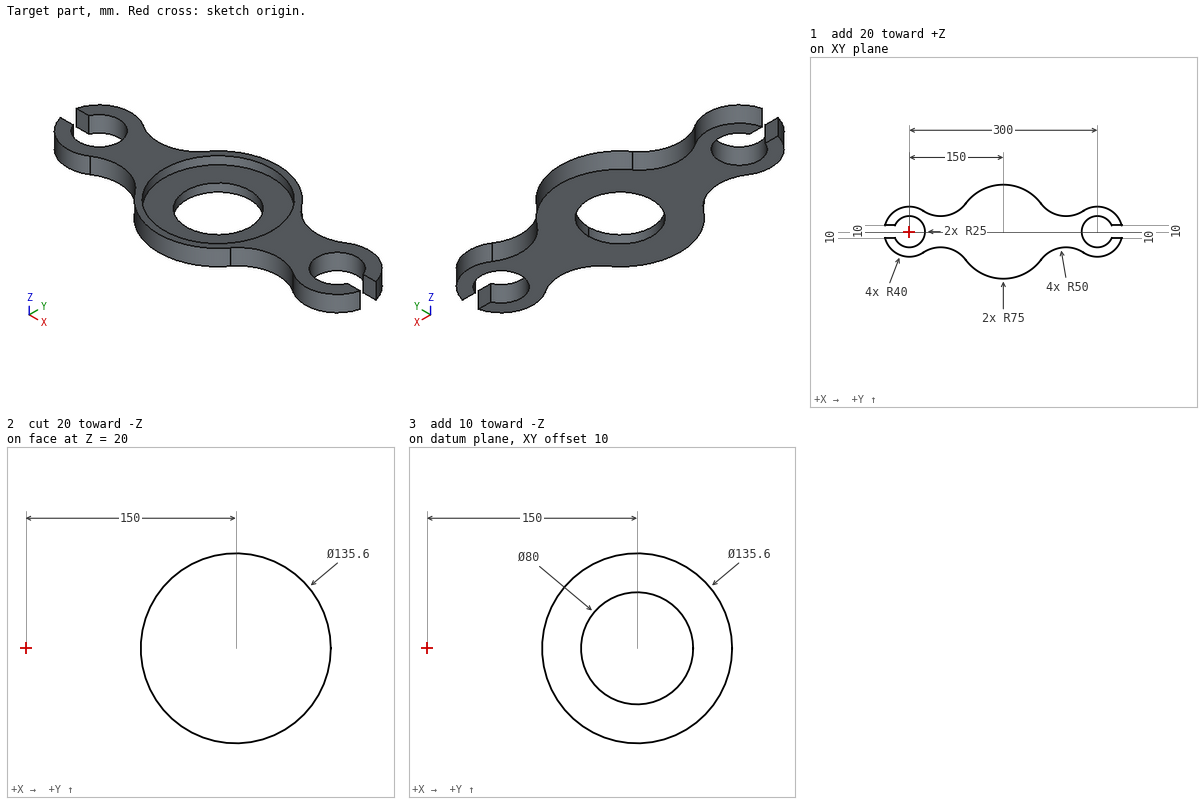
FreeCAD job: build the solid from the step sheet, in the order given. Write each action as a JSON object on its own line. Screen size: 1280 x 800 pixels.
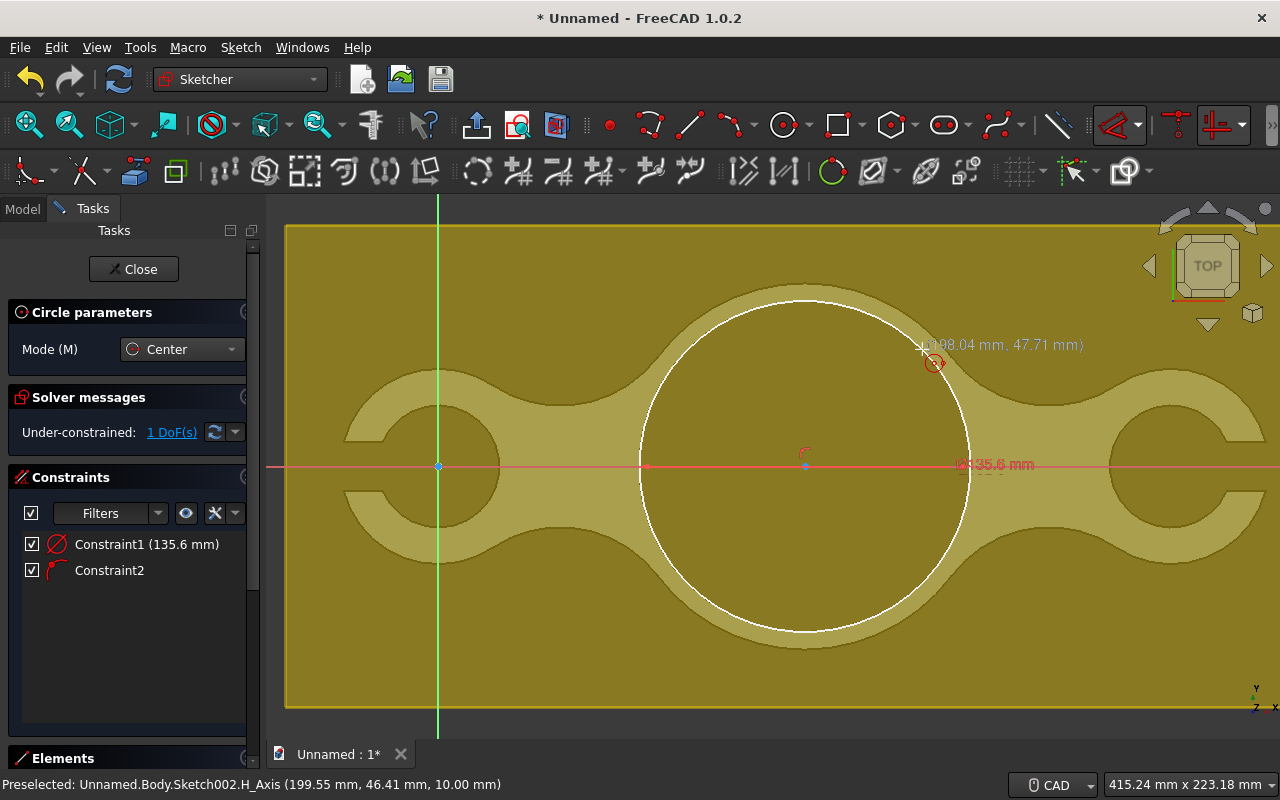
{"action": "left_click", "coordinate": [805, 466]}
{"action": "mouse_move", "coordinate": [874, 397]}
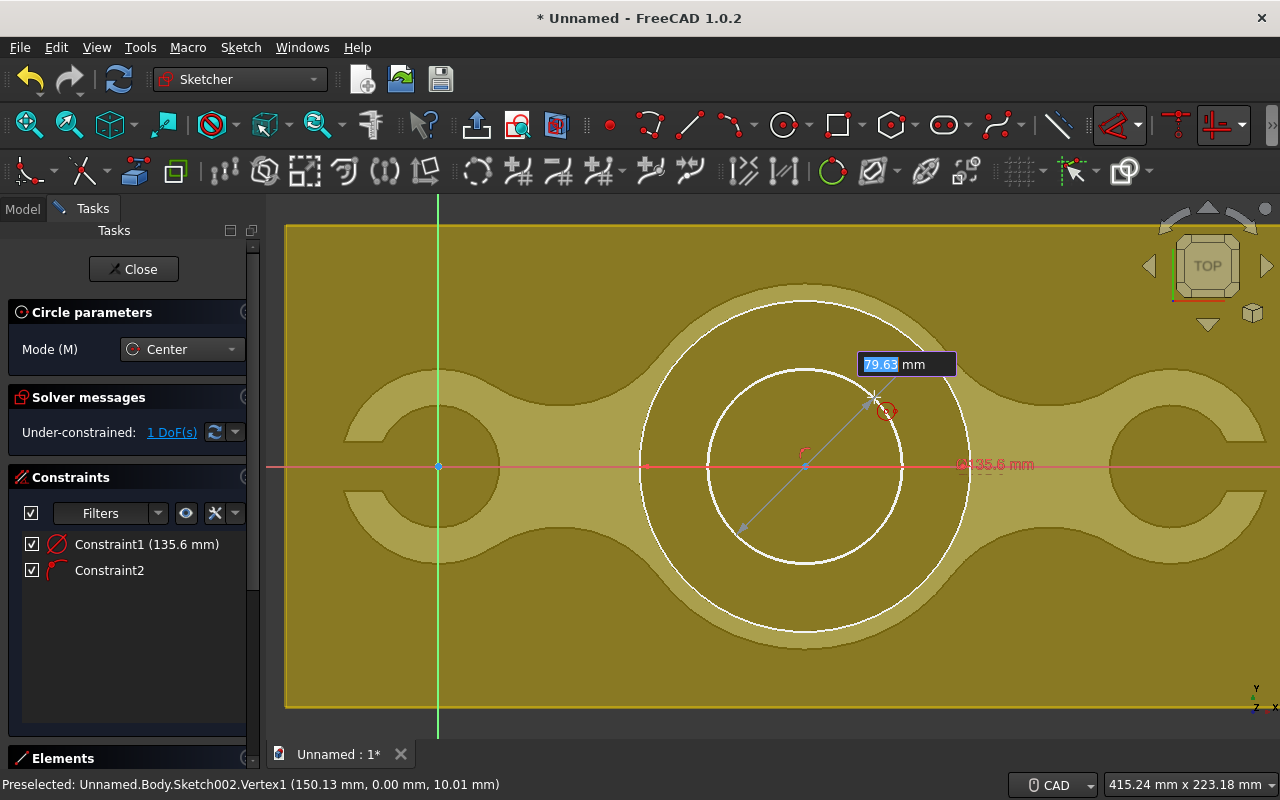
{"action": "type", "text": "80"}
{"action": "key", "text": "Return"}
{"action": "key", "text": "Escape"}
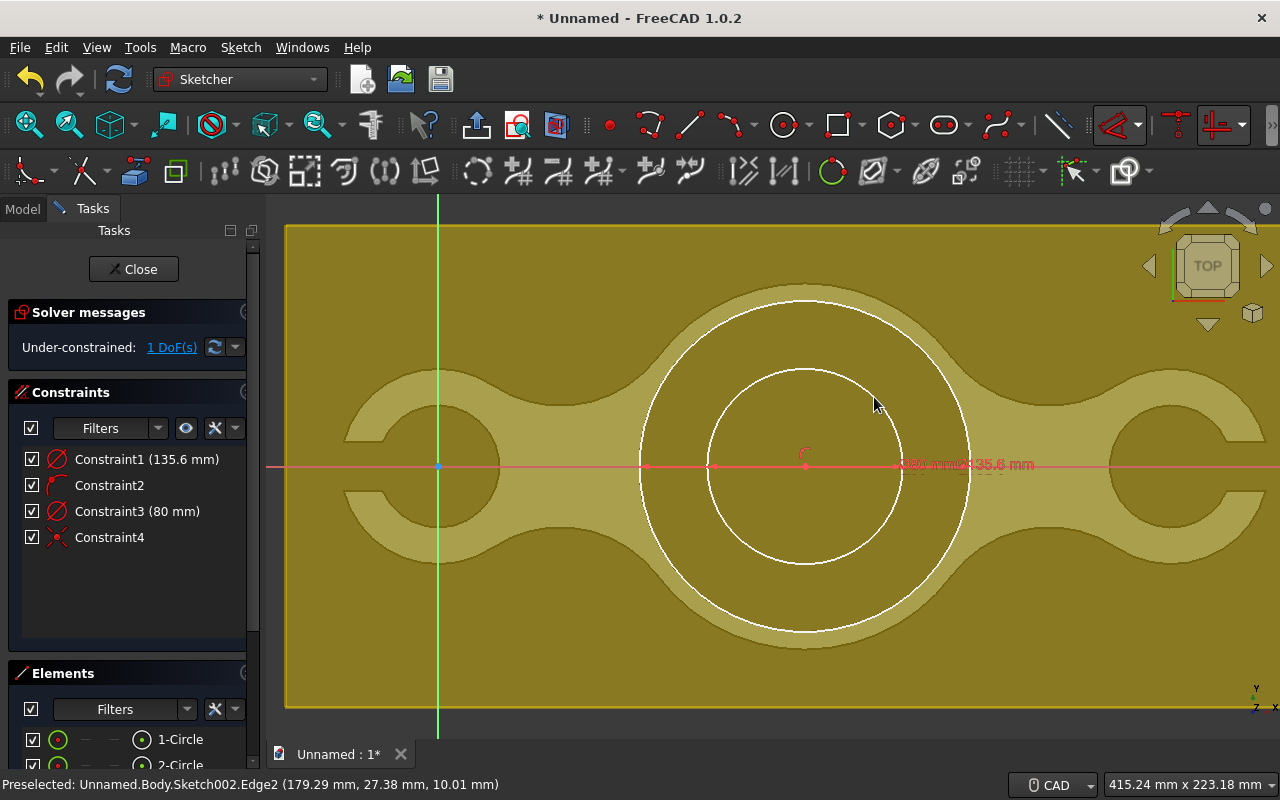
{"action": "left_click", "coordinate": [805, 466]}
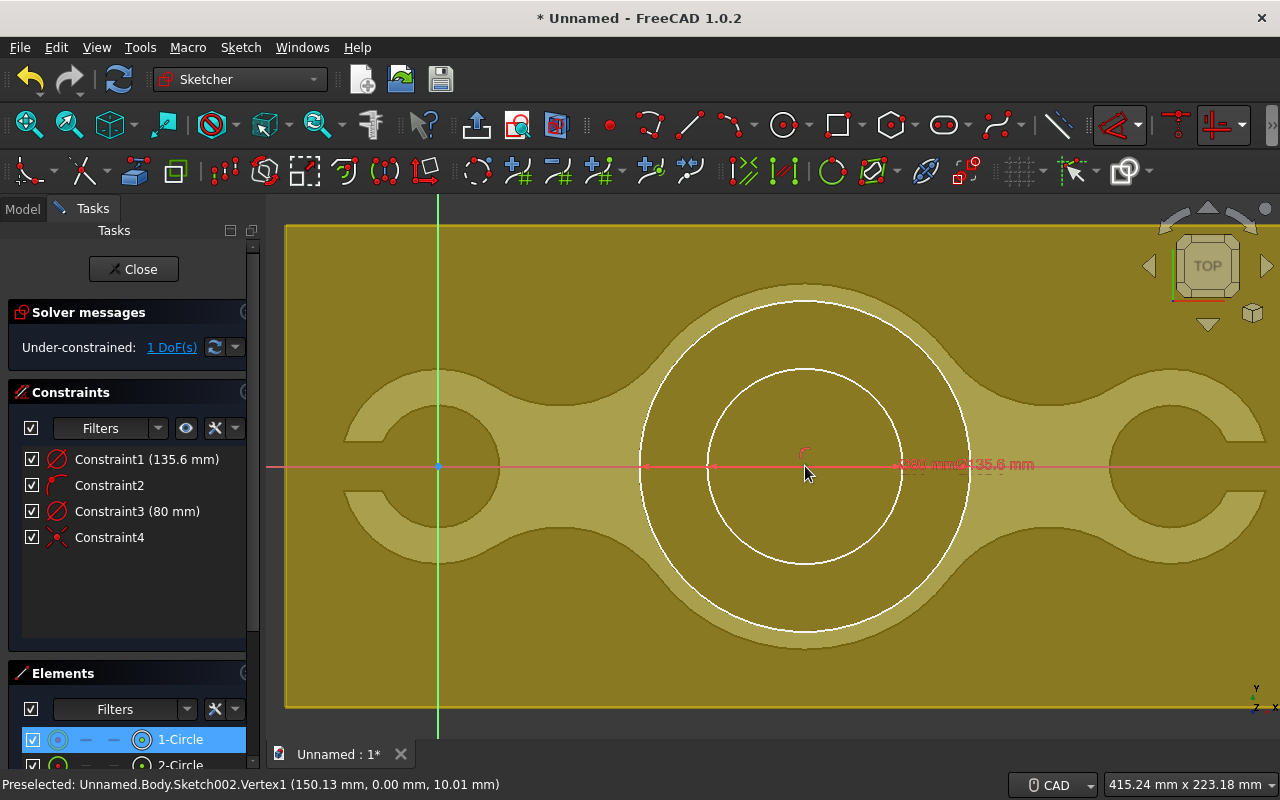
{"action": "key", "text": "l"}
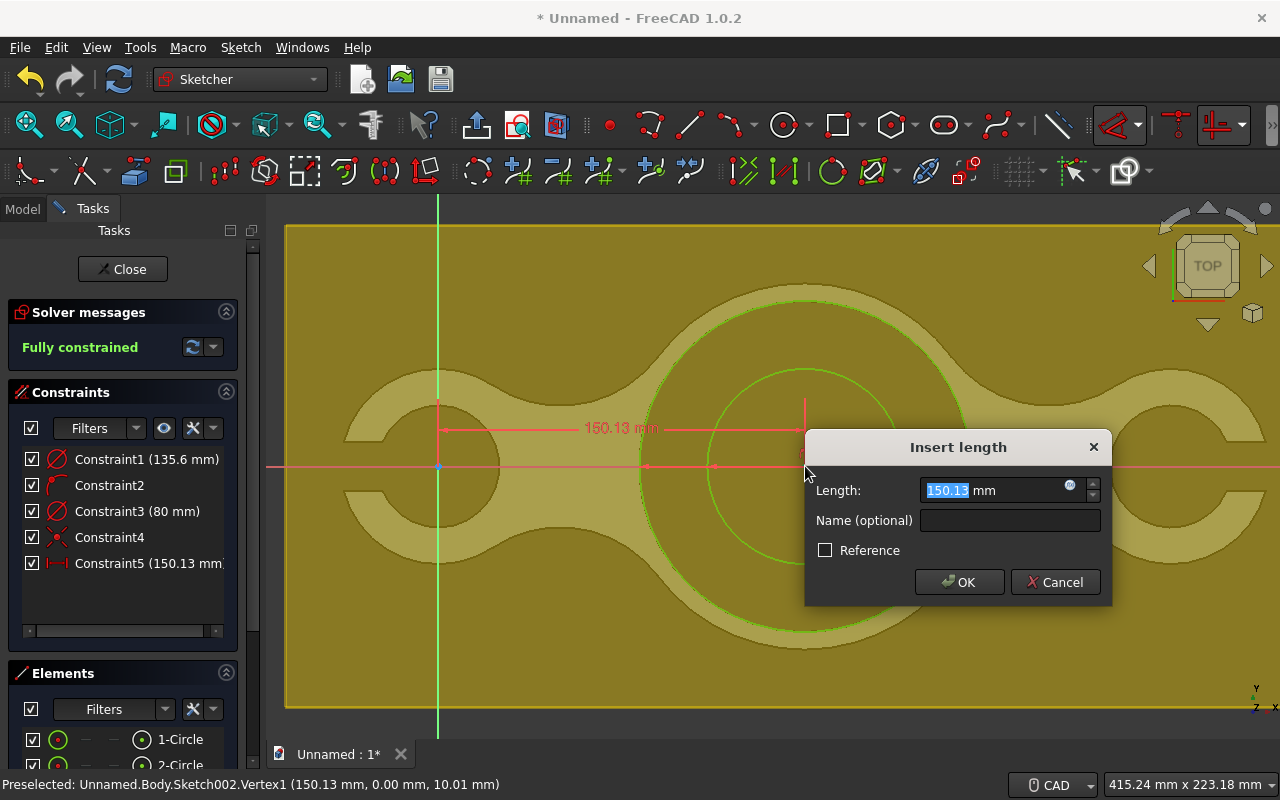
{"action": "type", "text": "150"}
{"action": "key", "text": "Return"}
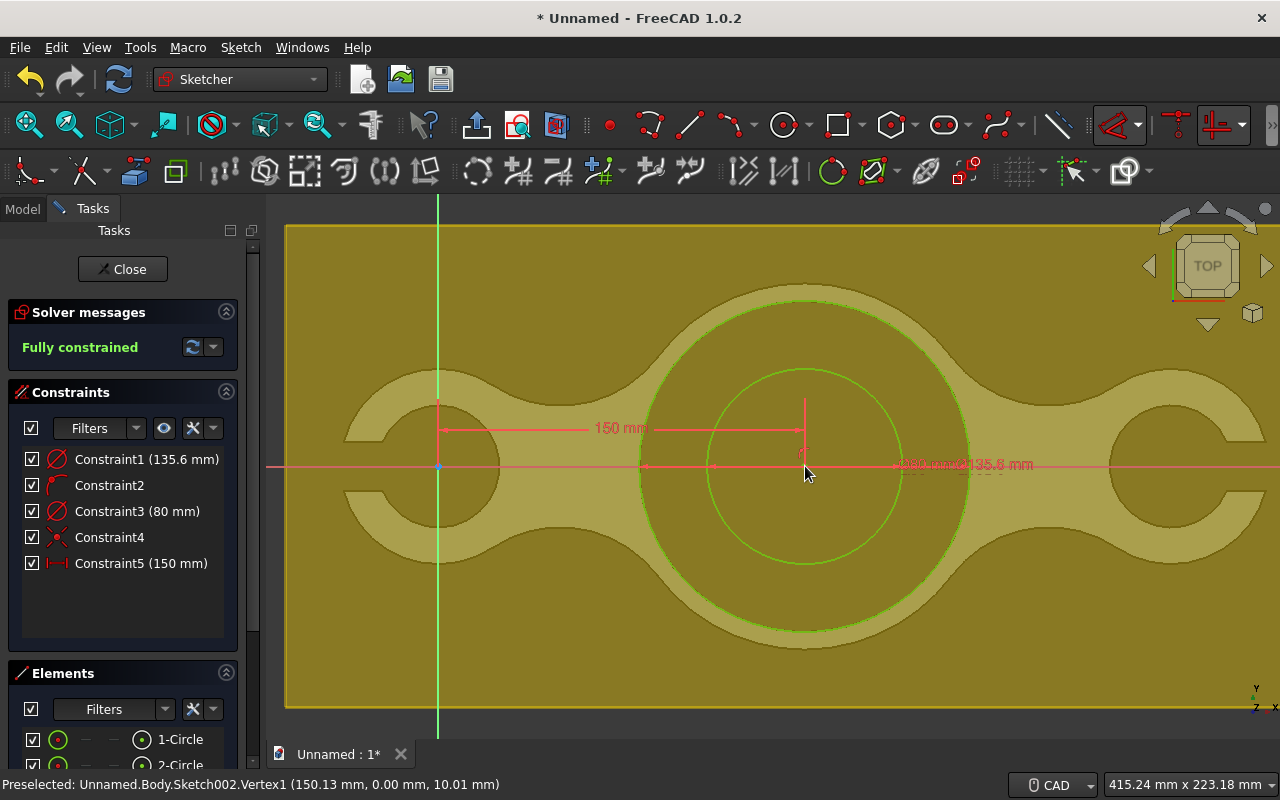
{"action": "left_click", "coordinate": [123, 269]}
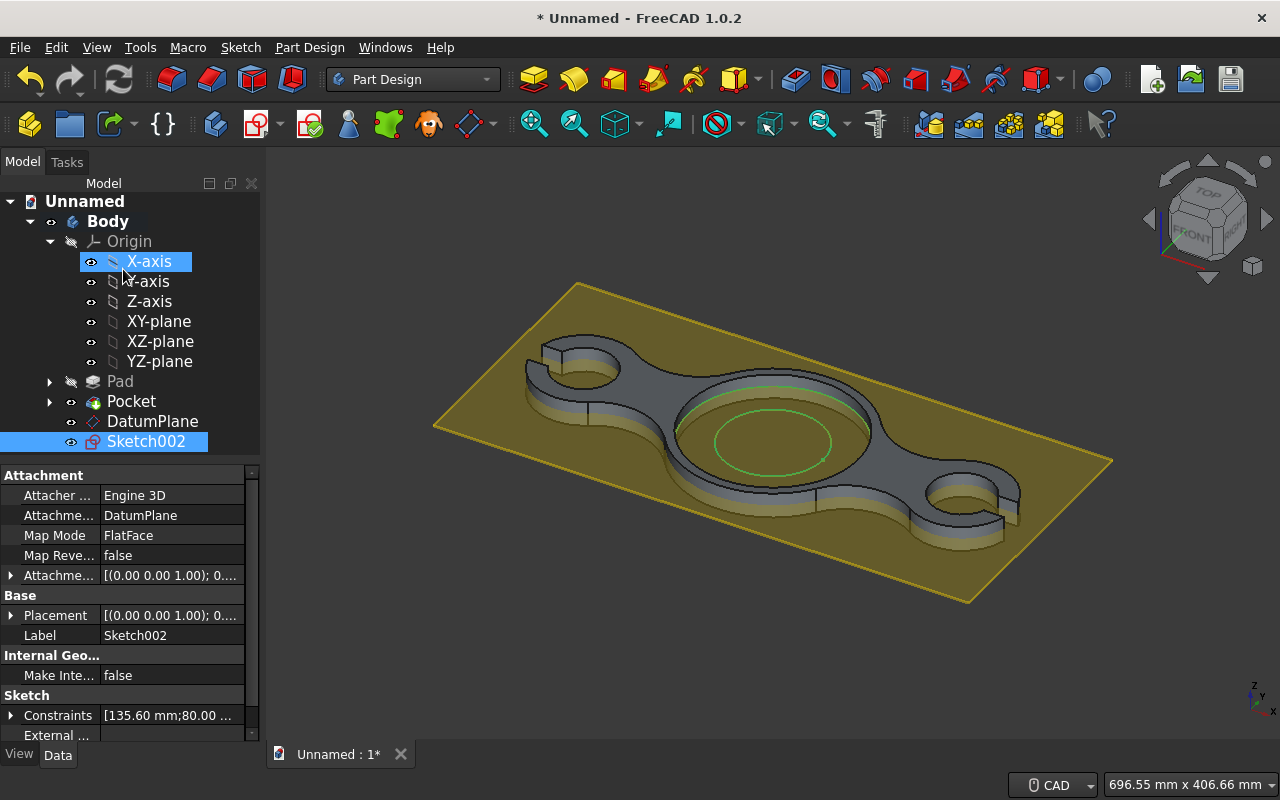
{"action": "left_click", "coordinate": [534, 80]}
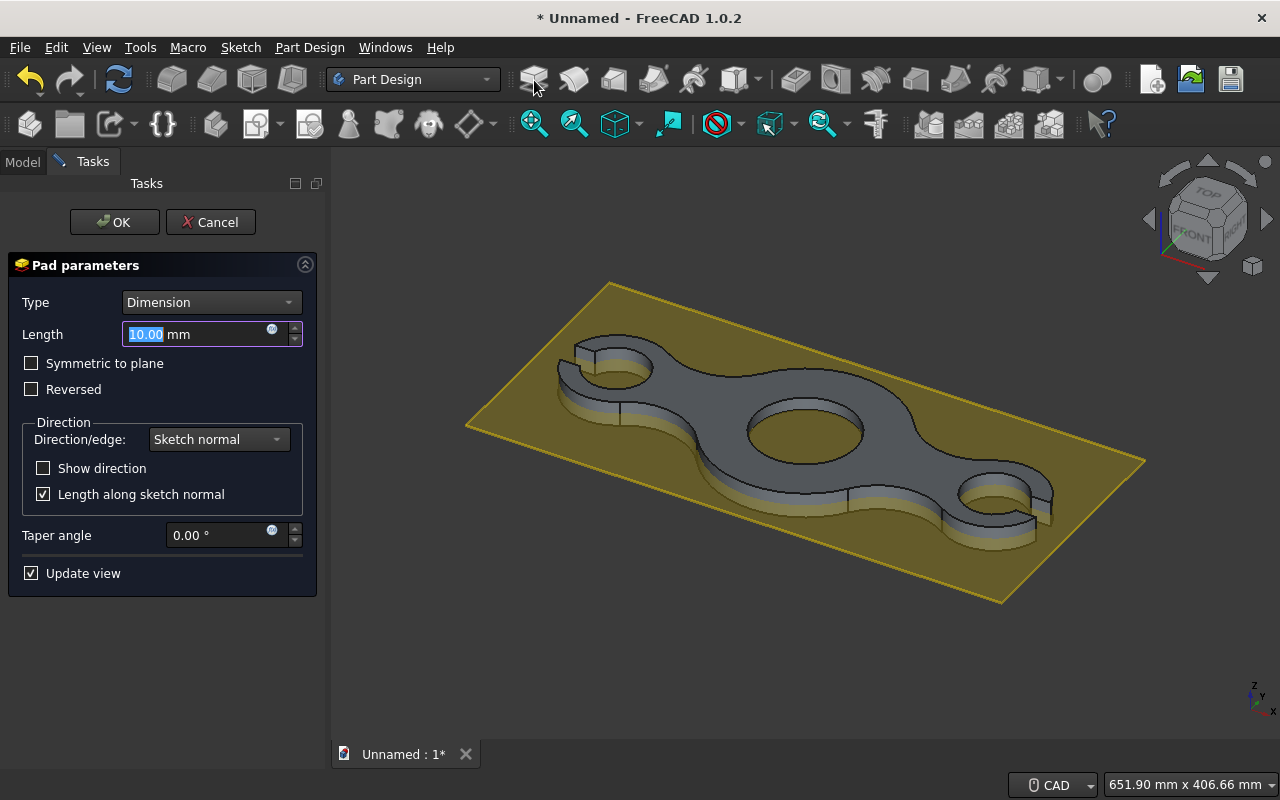
{"action": "type", "text": "10"}
{"action": "key", "text": "Tab"}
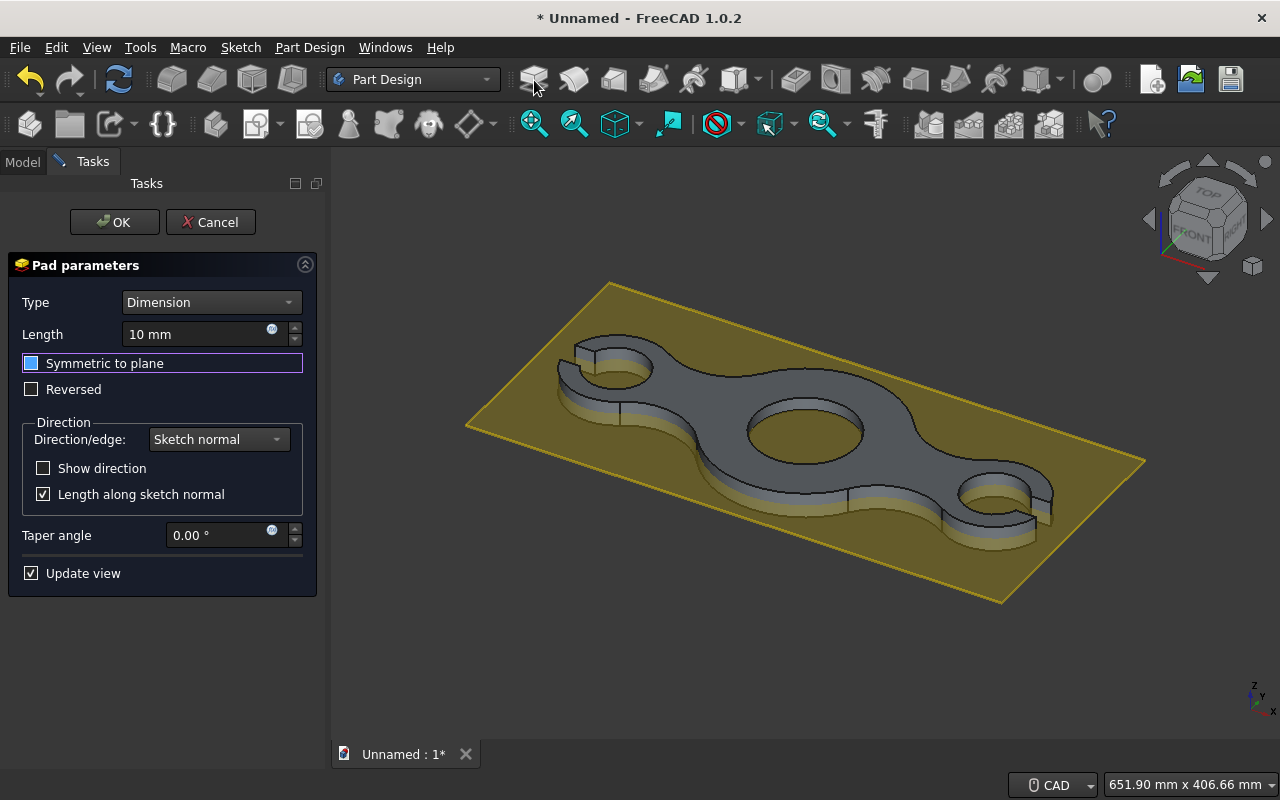
{"action": "left_click", "coordinate": [30, 389]}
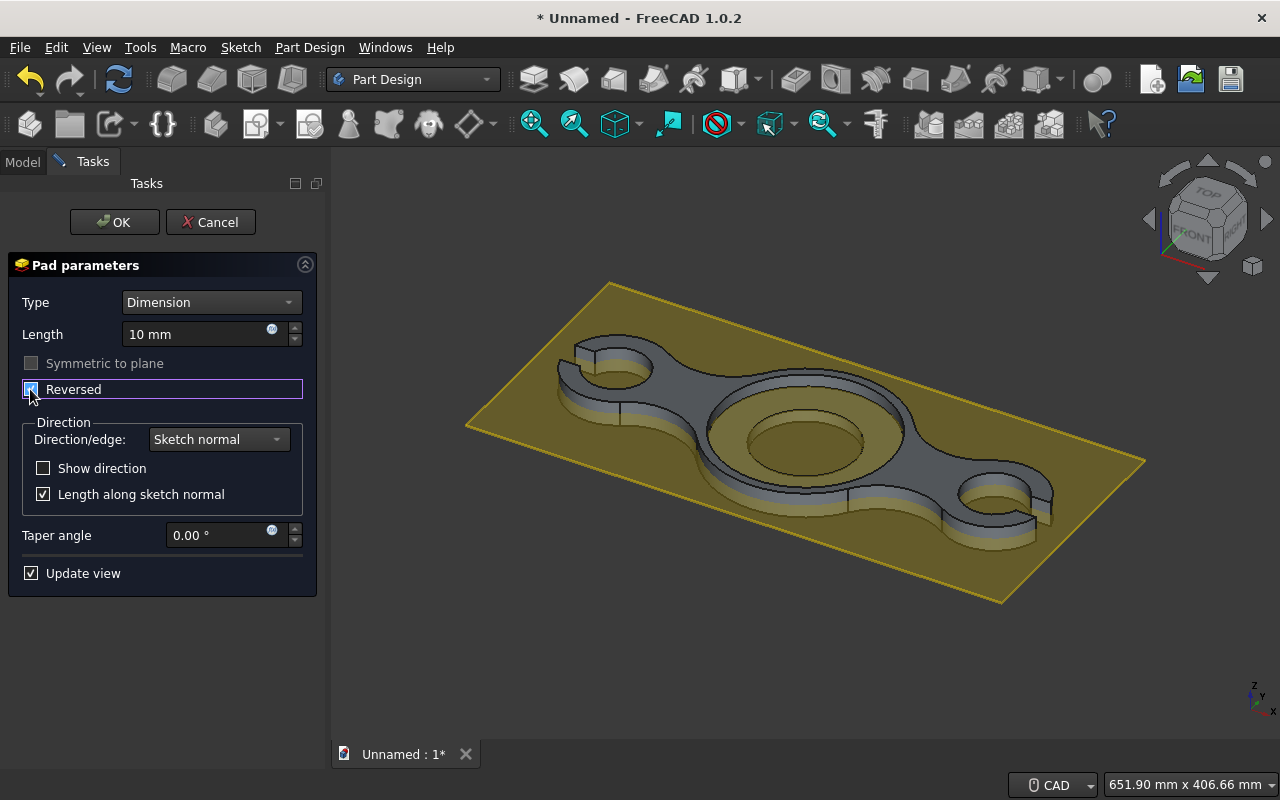
{"action": "left_click", "coordinate": [115, 222]}